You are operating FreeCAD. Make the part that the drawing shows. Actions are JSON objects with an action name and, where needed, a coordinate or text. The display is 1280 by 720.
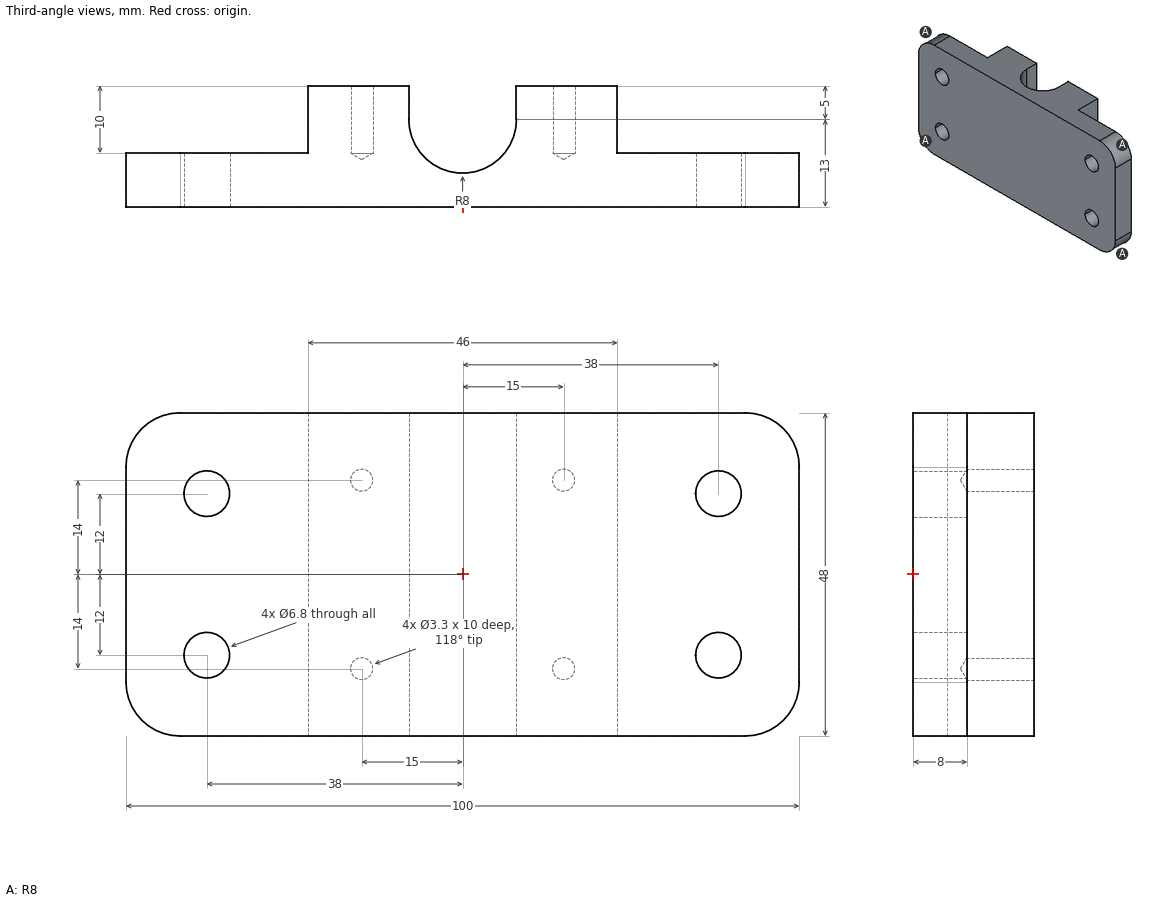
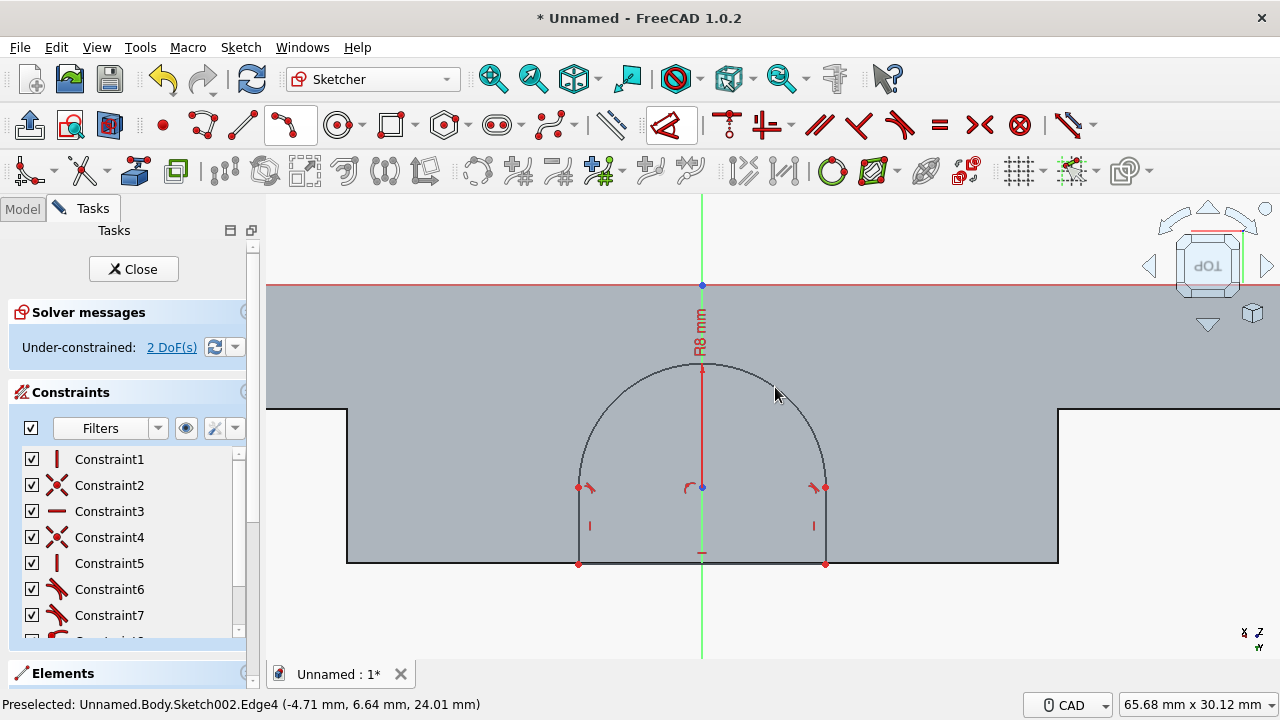
{"action": "left_click", "coordinate": [579, 510]}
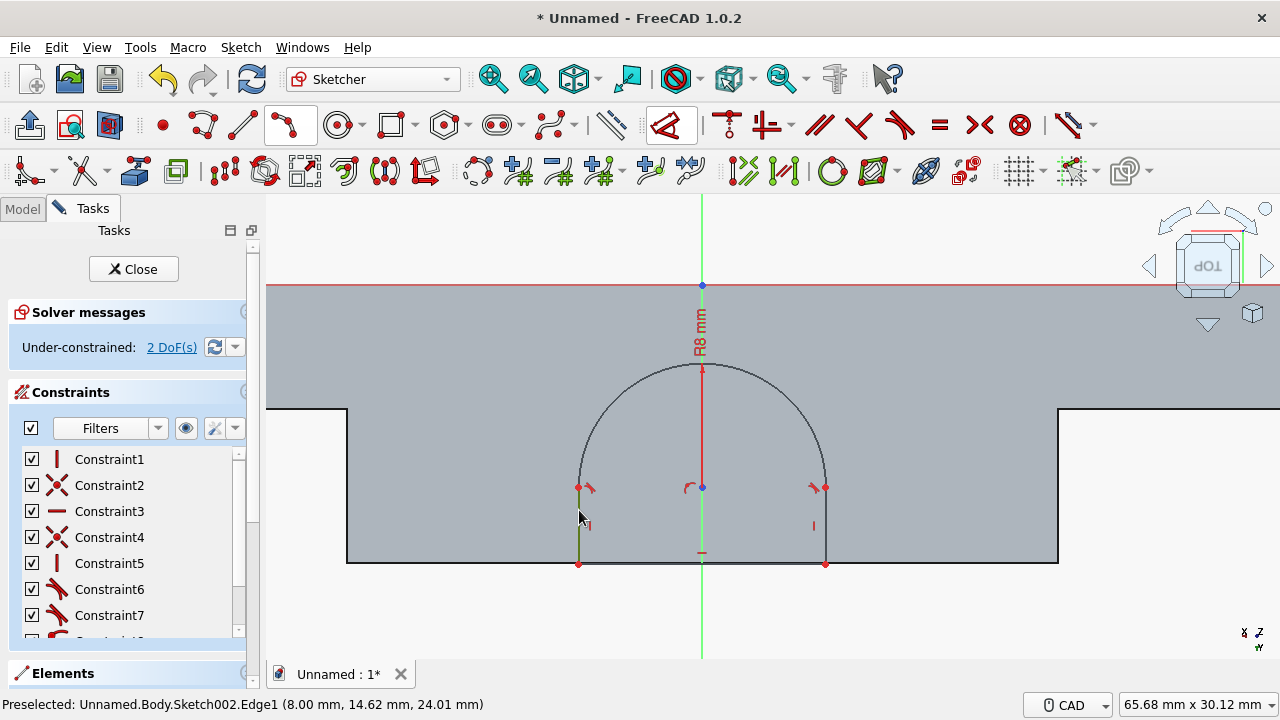
{"action": "left_click", "coordinate": [692, 126]}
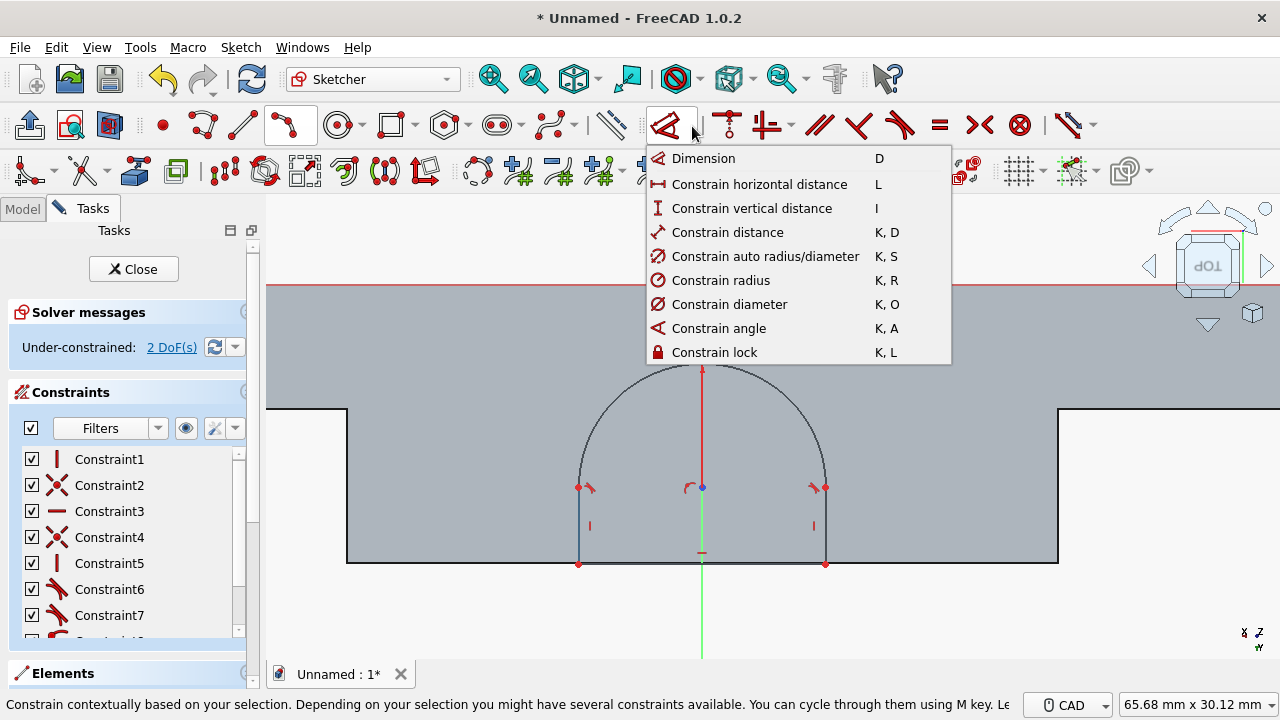
{"action": "left_click", "coordinate": [799, 208]}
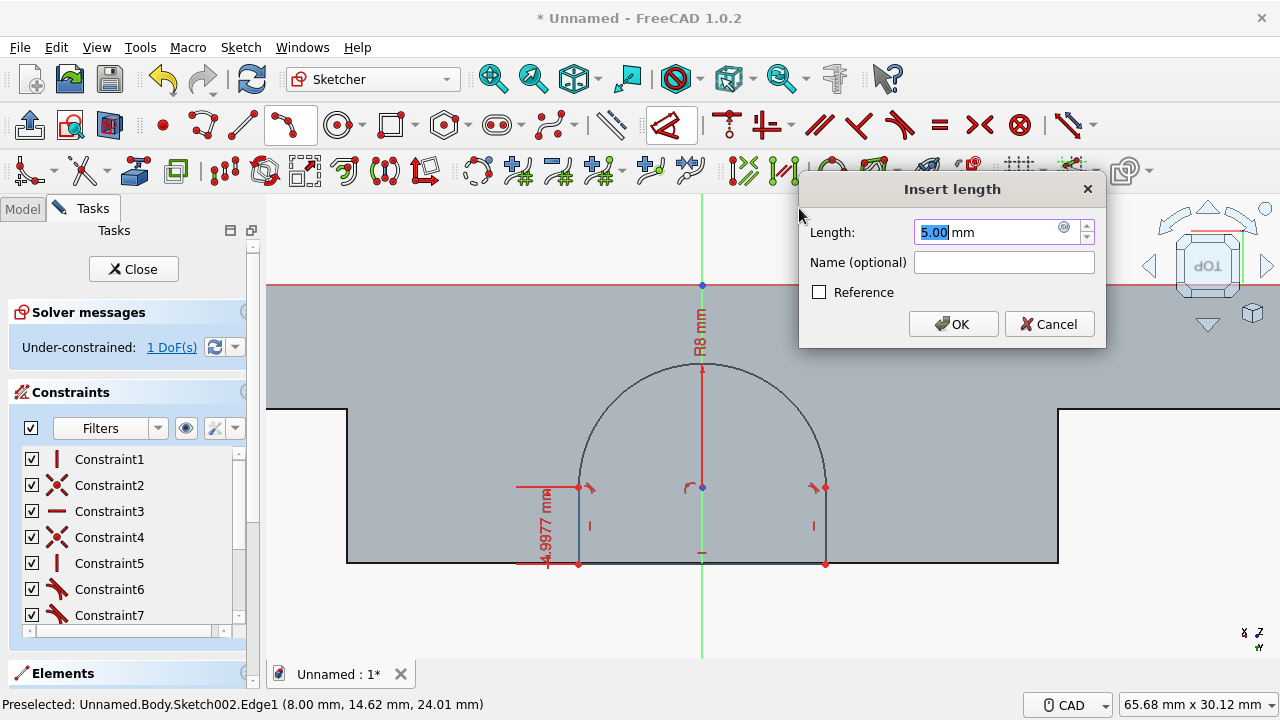
{"action": "type", "text": "5"}
{"action": "key", "text": "Return"}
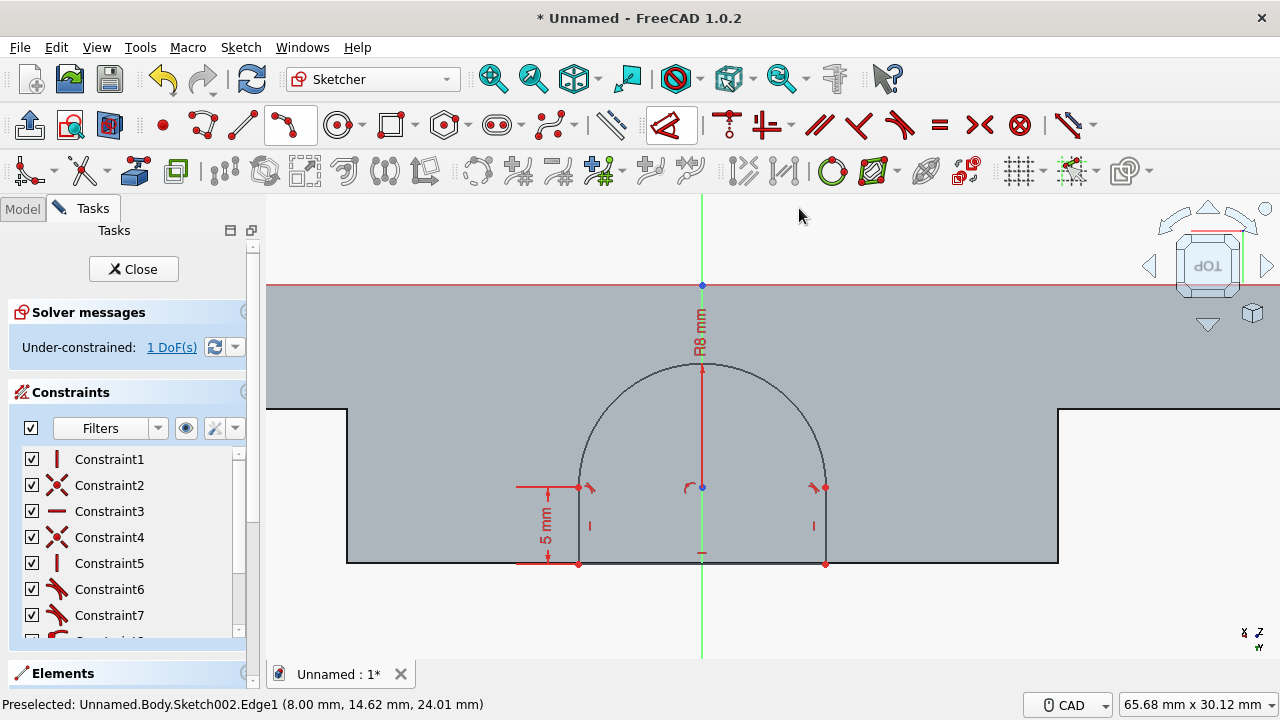
{"action": "left_click", "coordinate": [579, 487]}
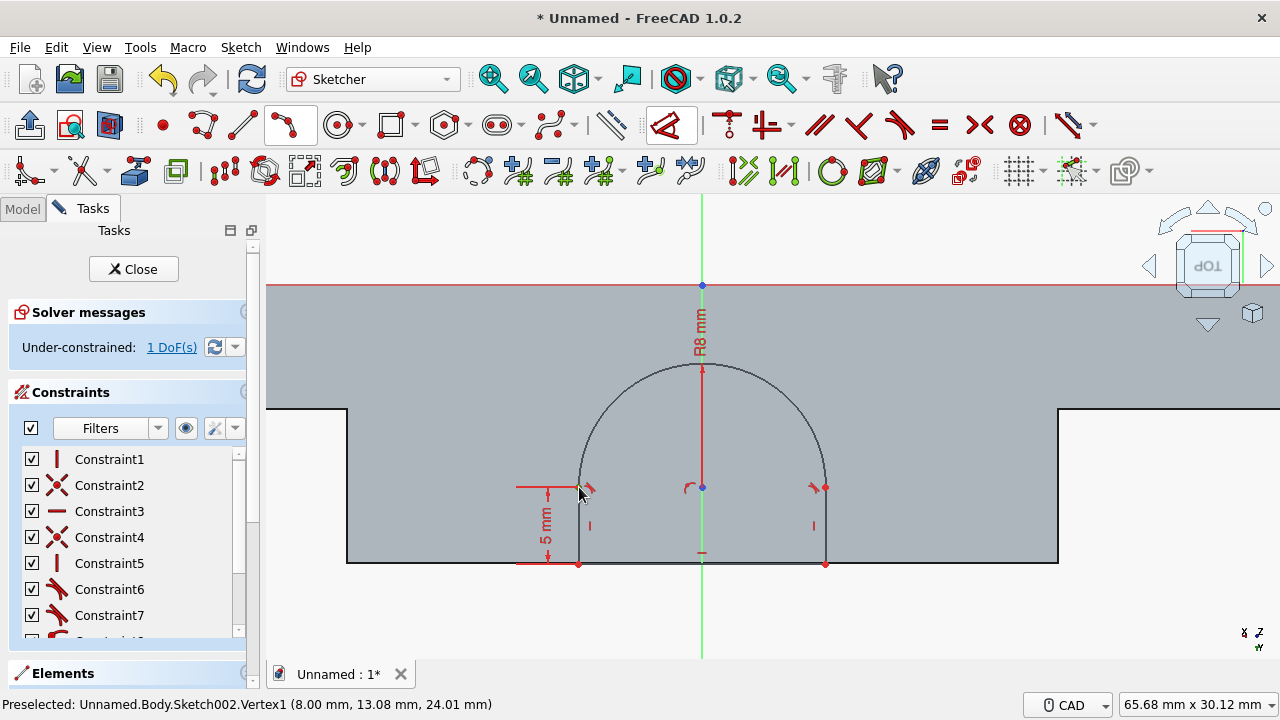
{"action": "key", "text": "i"}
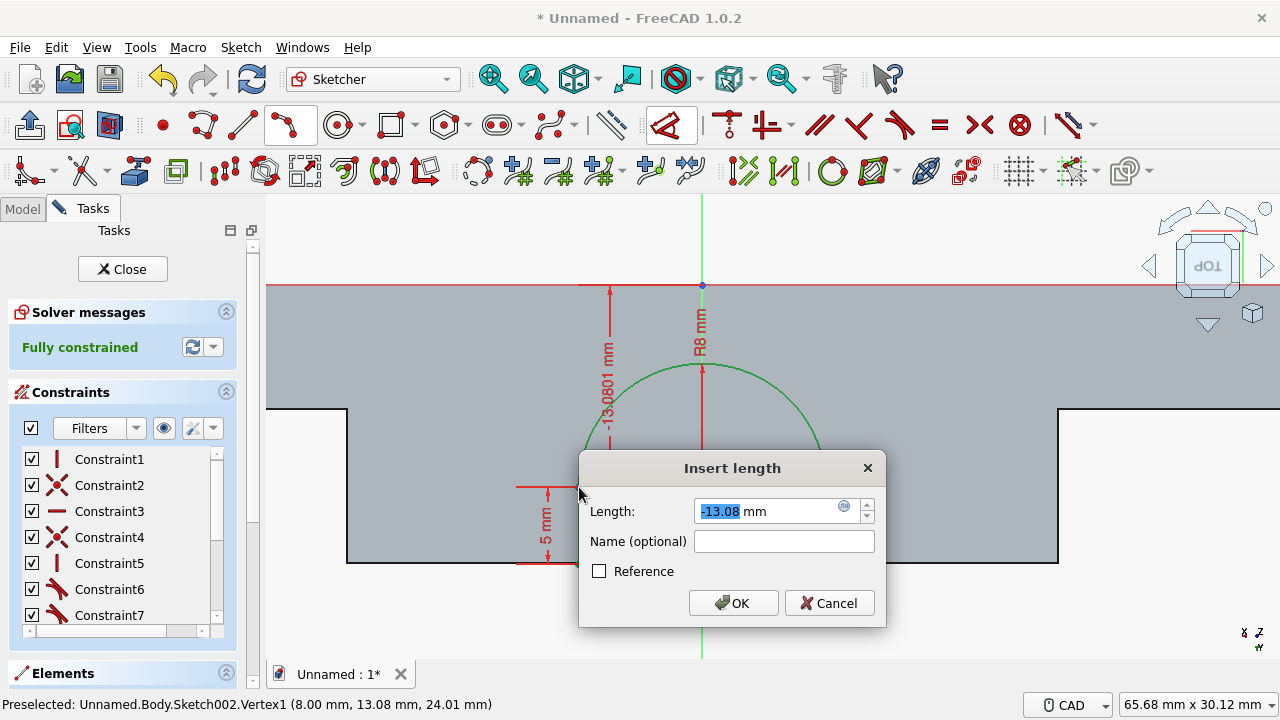
{"action": "type", "text": "-13"}
{"action": "key", "text": "Return"}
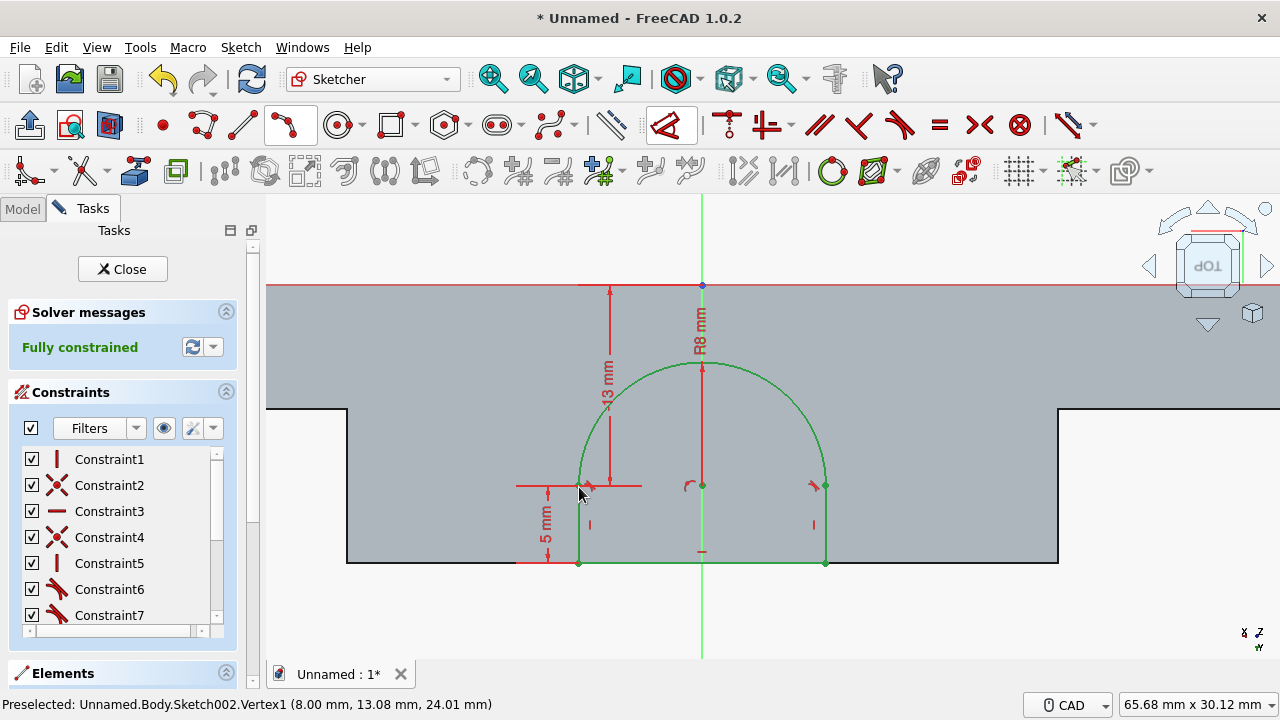
{"action": "left_click", "coordinate": [123, 269]}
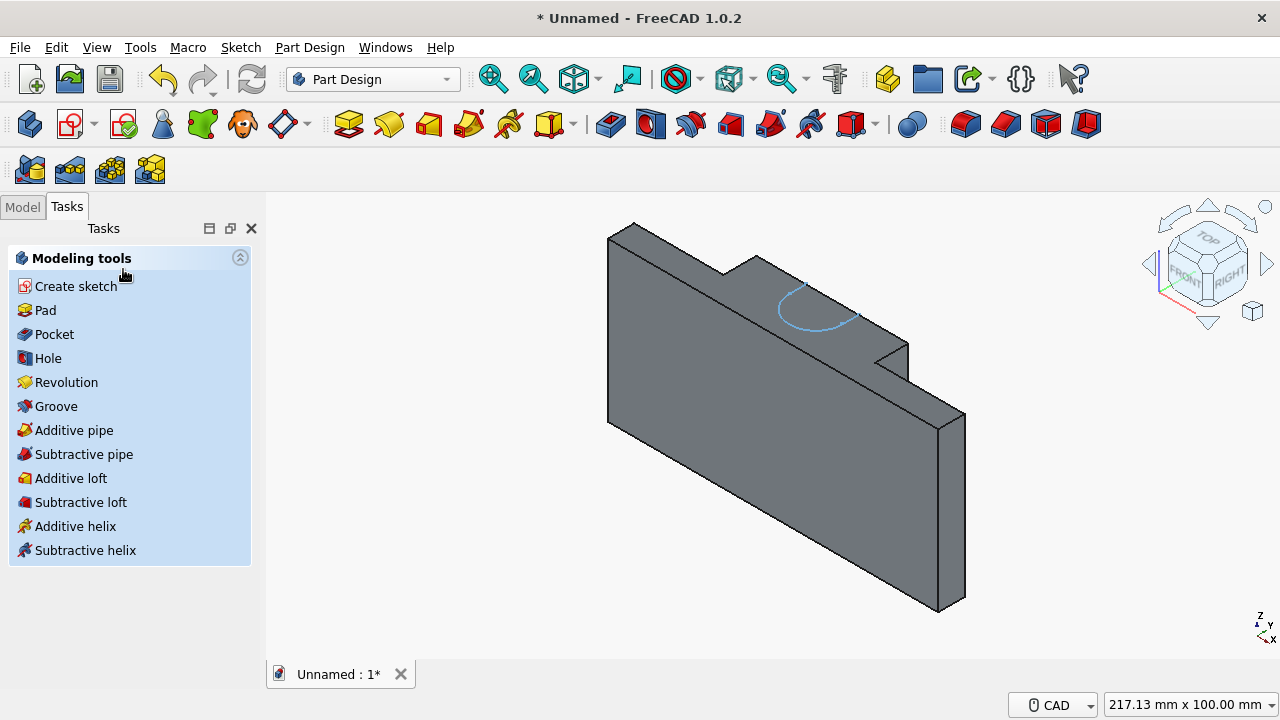
{"action": "left_click", "coordinate": [612, 124]}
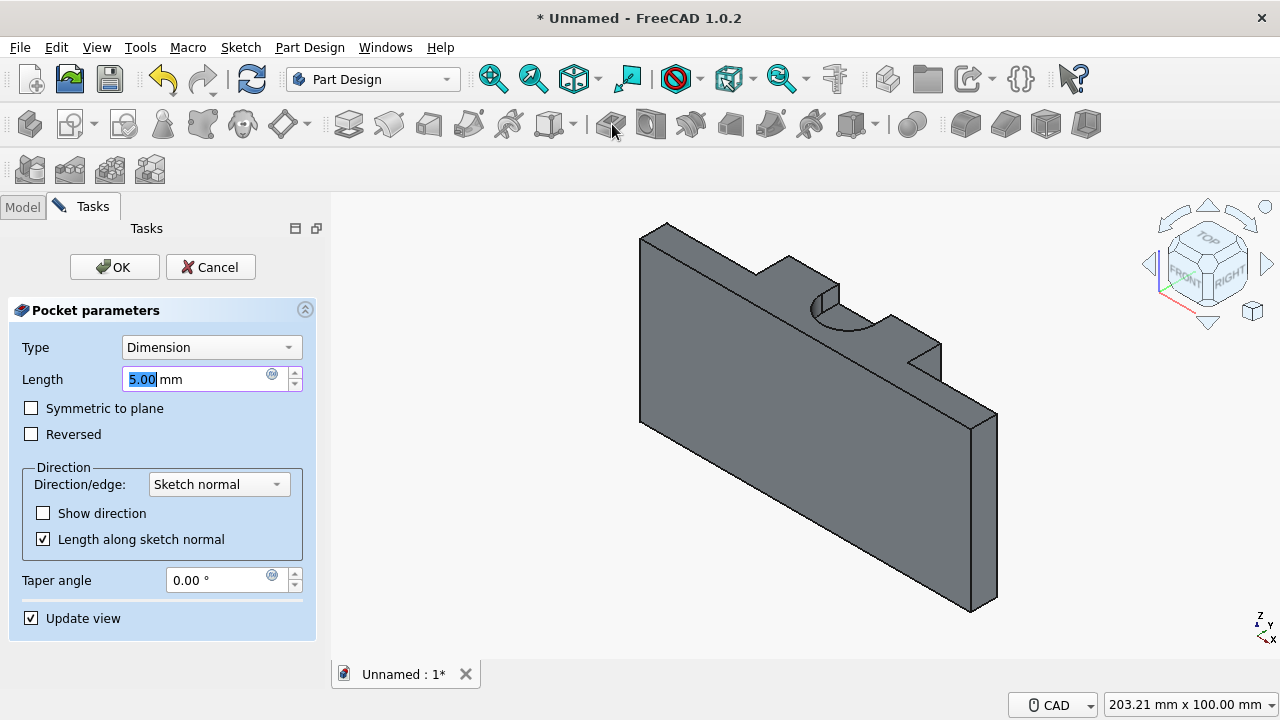
{"action": "left_click", "coordinate": [212, 348]}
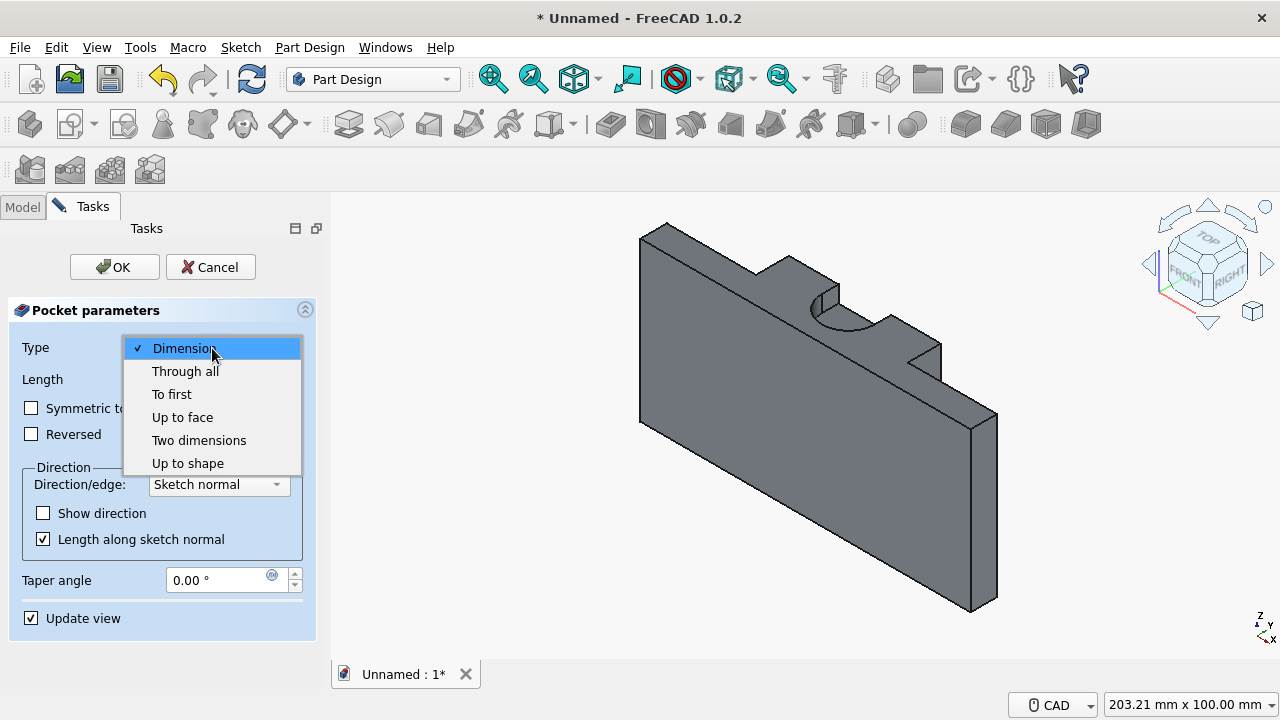
{"action": "left_click", "coordinate": [212, 372]}